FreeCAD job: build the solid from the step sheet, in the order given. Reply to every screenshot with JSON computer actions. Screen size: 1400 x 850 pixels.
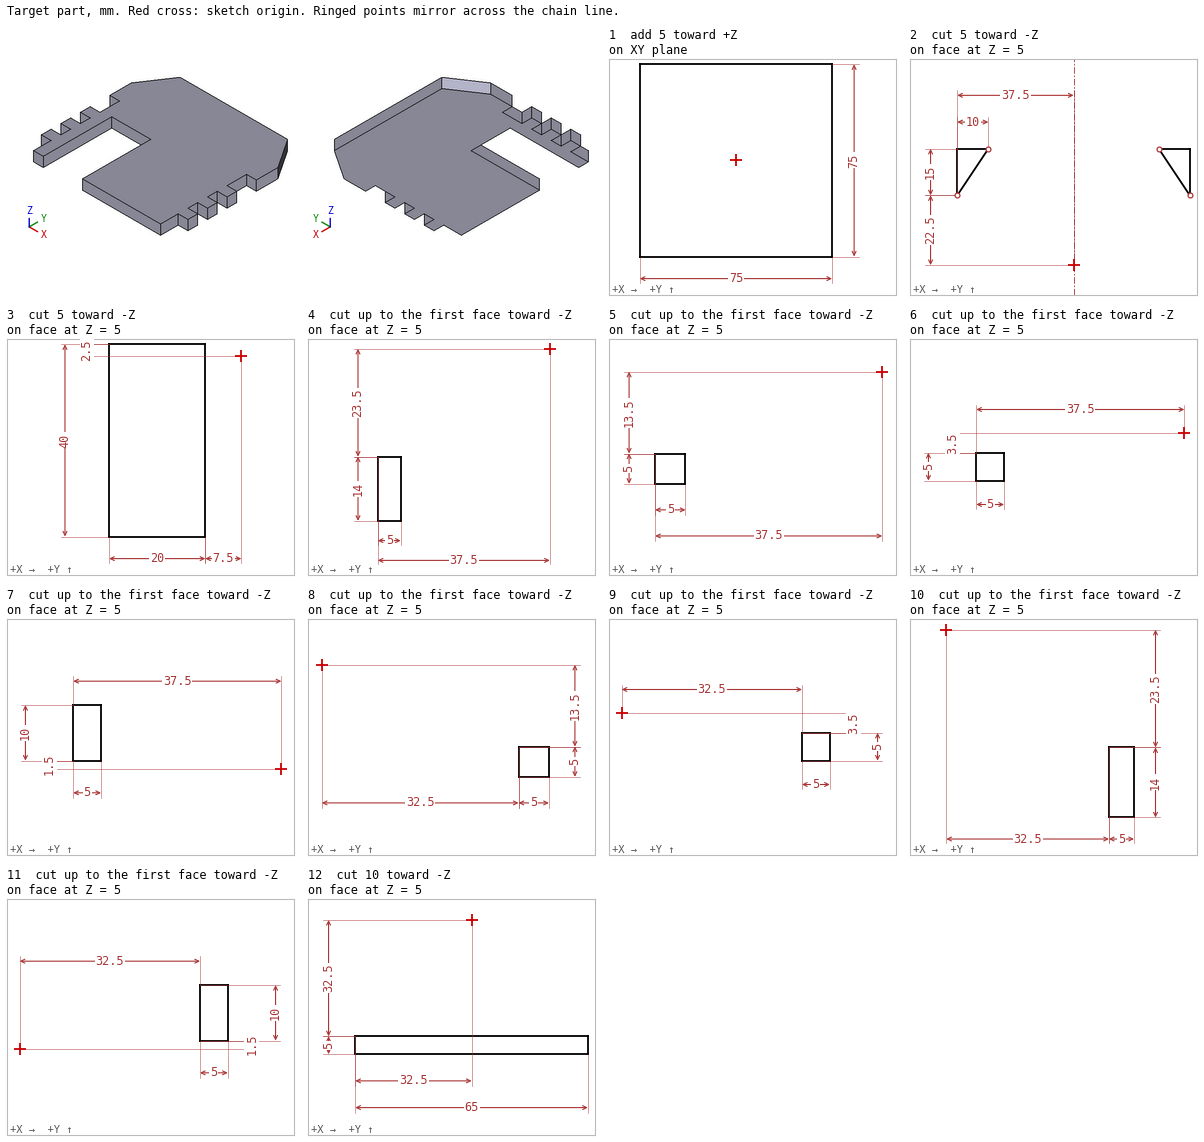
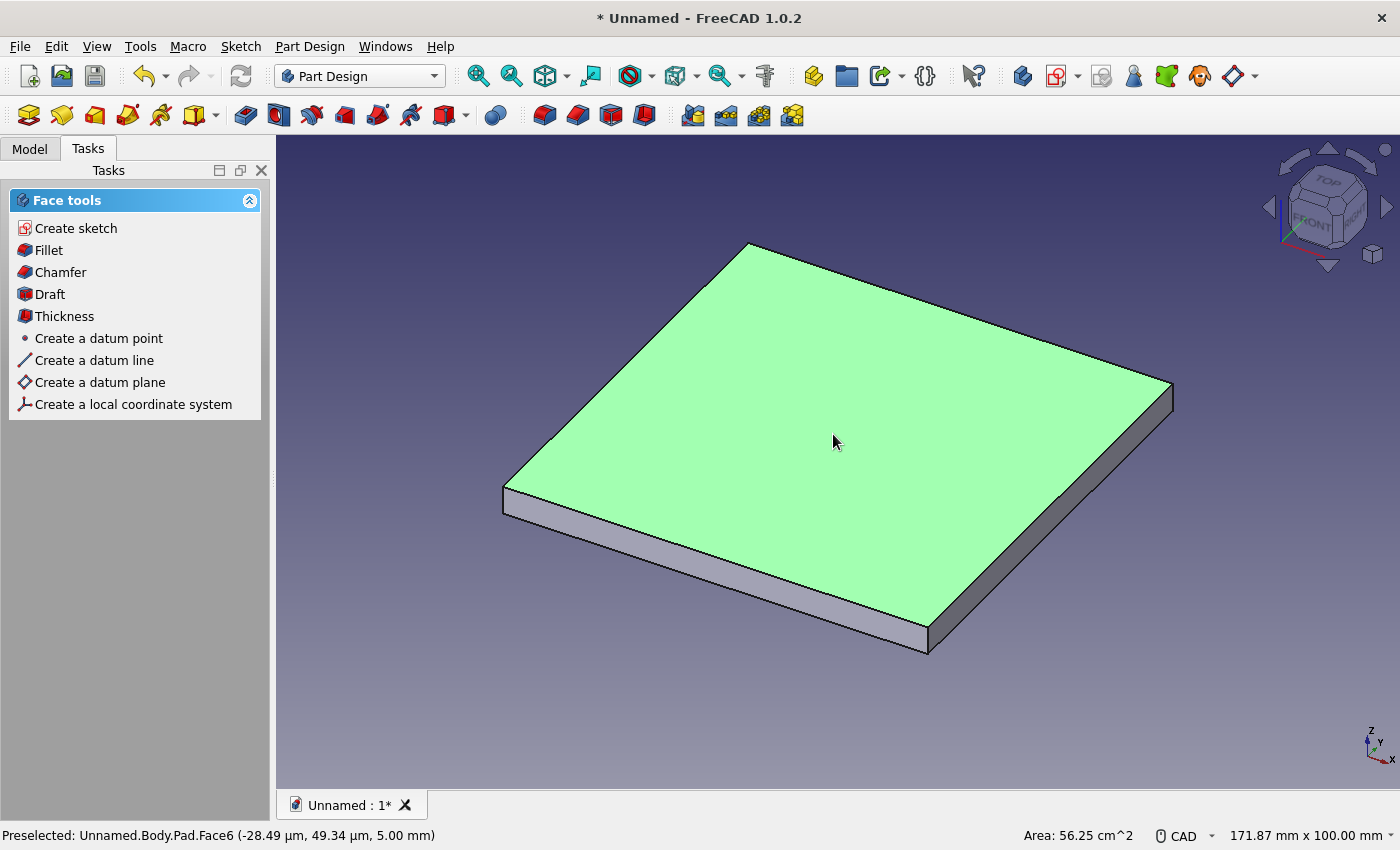
{"action": "left_click", "coordinate": [1056, 76]}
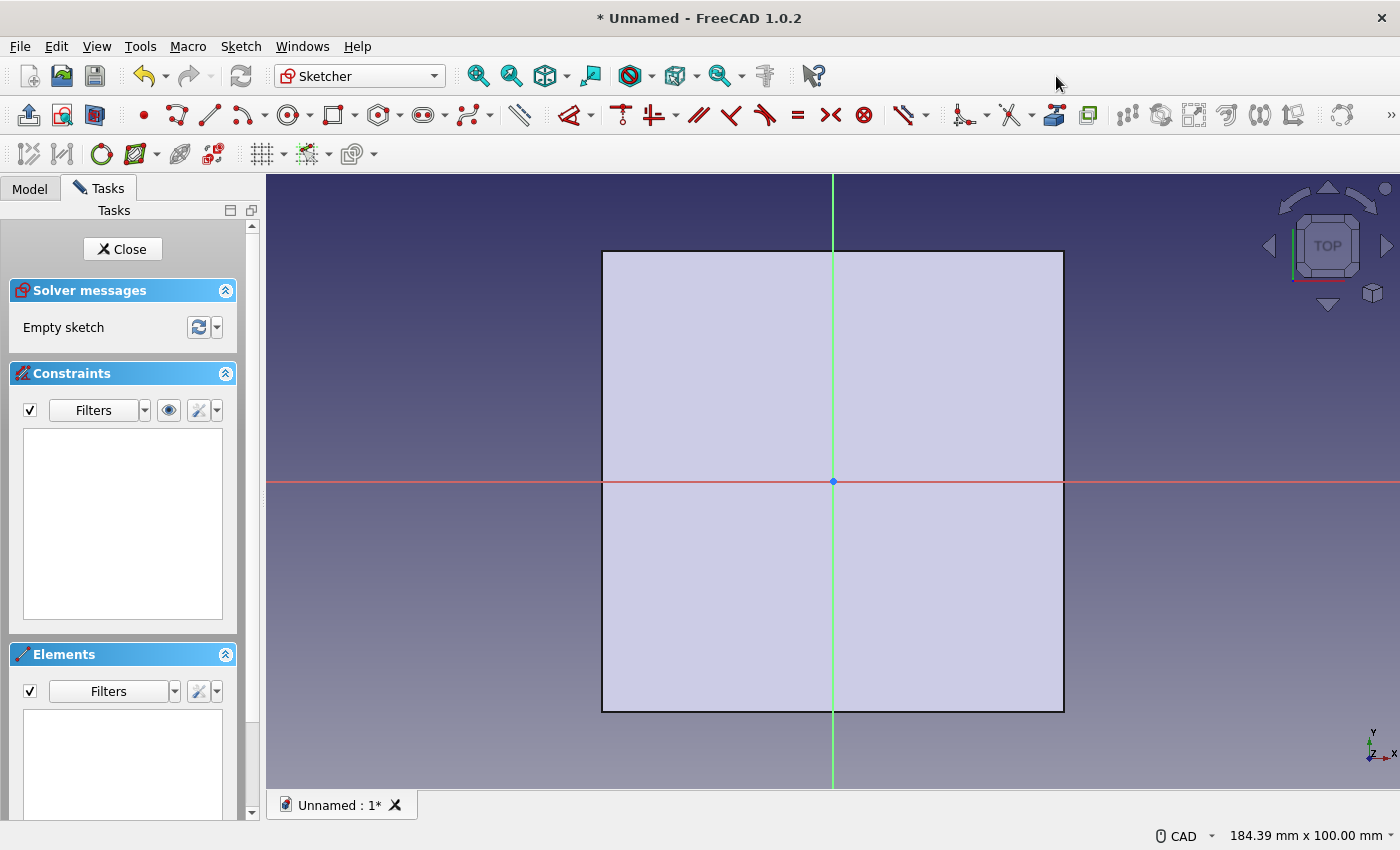
{"action": "scroll", "coordinate": [972, 202], "scroll_direction": "up", "scroll_amount": 2}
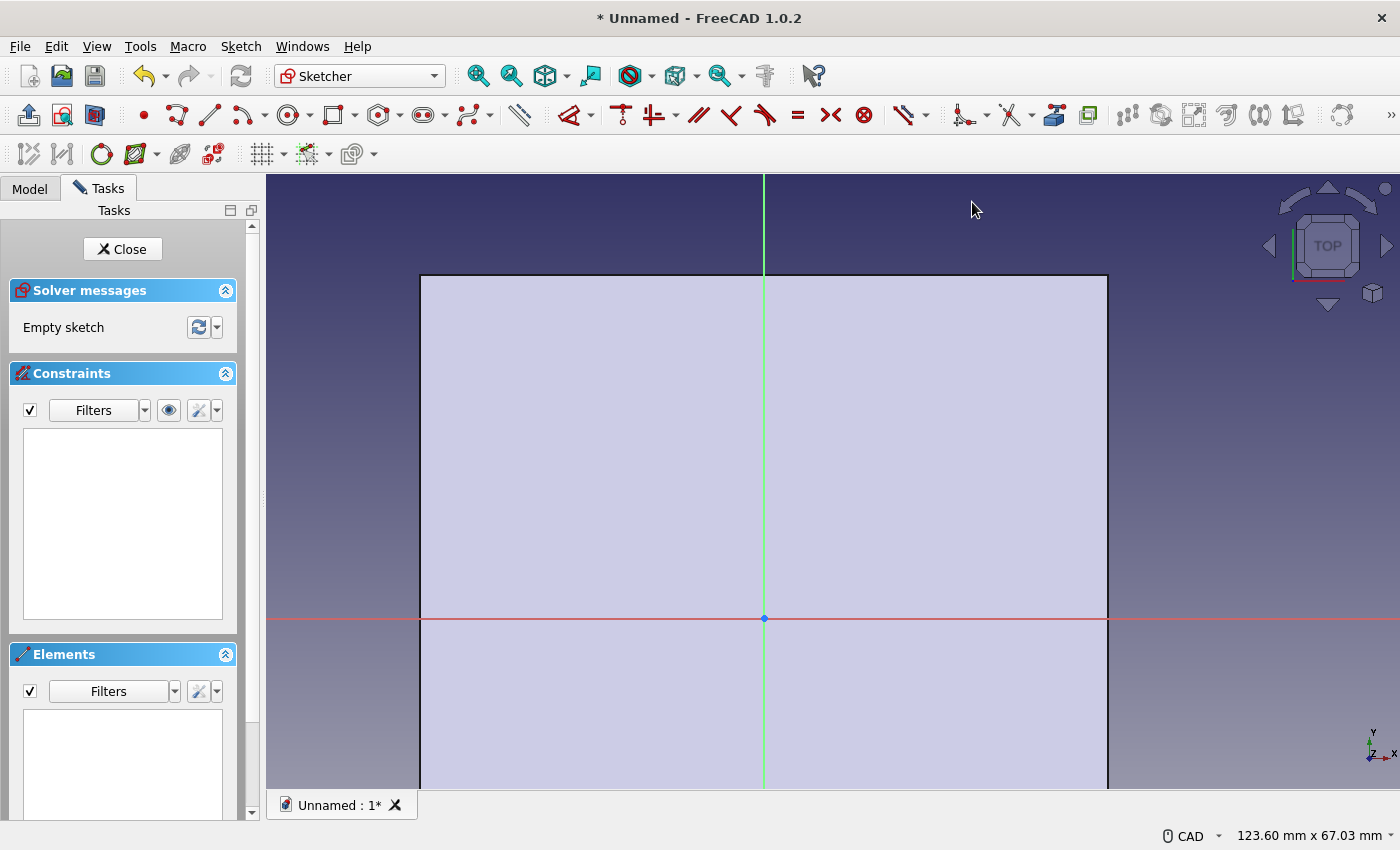
{"action": "left_click", "coordinate": [177, 116]}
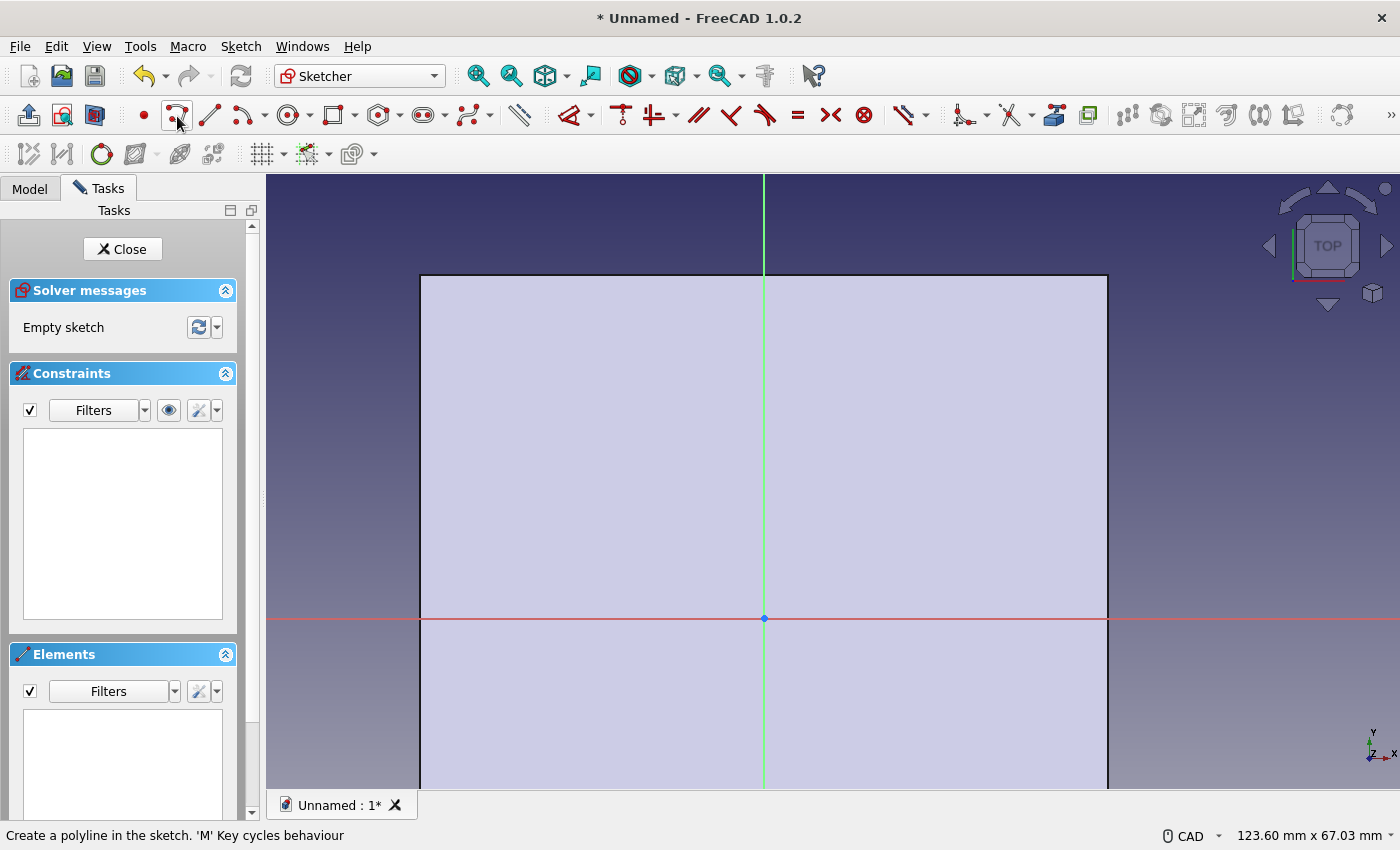
{"action": "left_click", "coordinate": [420, 413]}
{"action": "left_click", "coordinate": [512, 275]}
{"action": "left_click", "coordinate": [420, 275]}
{"action": "left_click", "coordinate": [420, 414]}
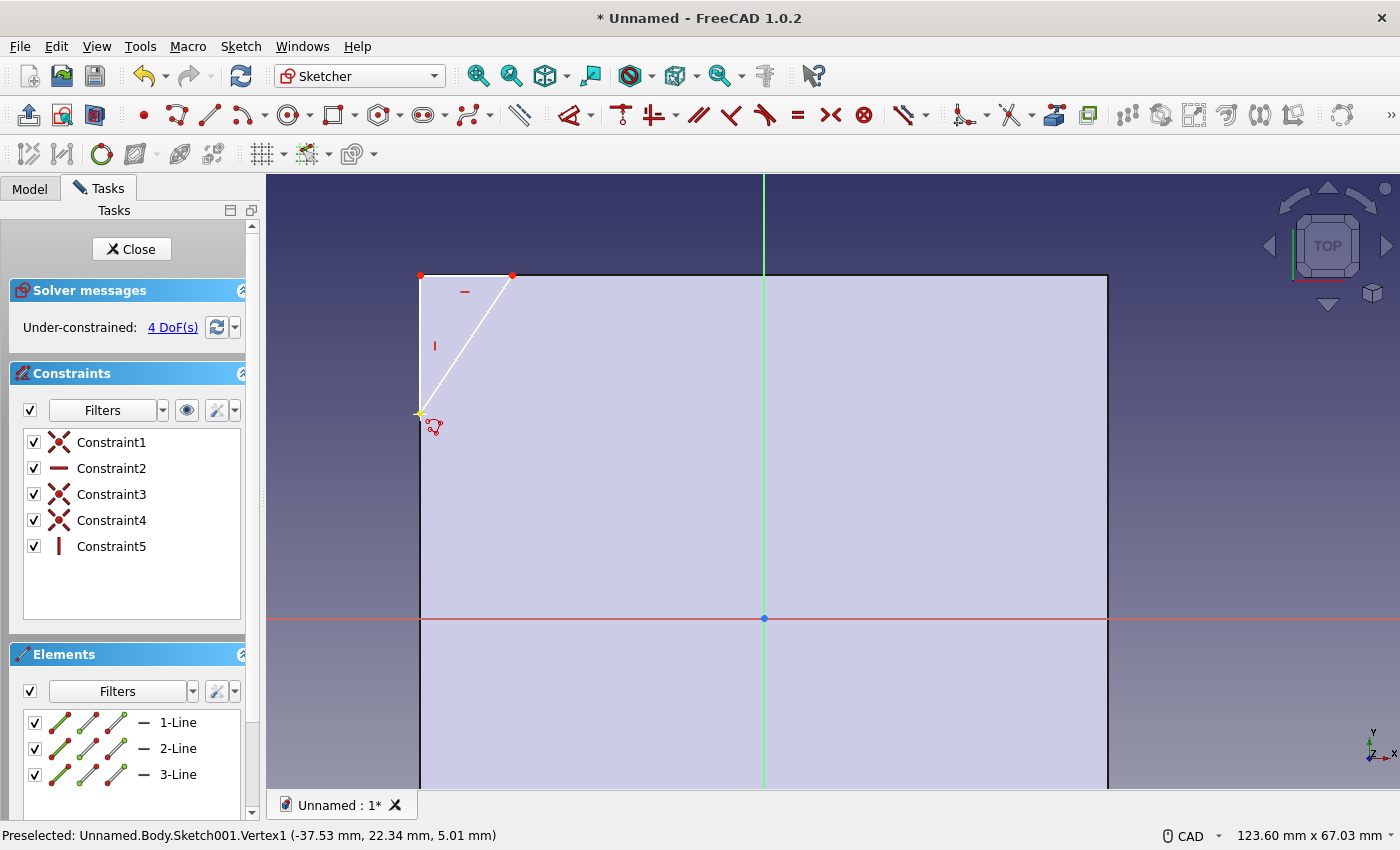
{"action": "left_click", "coordinate": [1108, 413]}
{"action": "left_click", "coordinate": [1108, 275]}
{"action": "left_click", "coordinate": [1017, 275]}
{"action": "left_click", "coordinate": [1108, 414]}
{"action": "key", "text": "Escape"}
{"action": "key", "text": "Escape"}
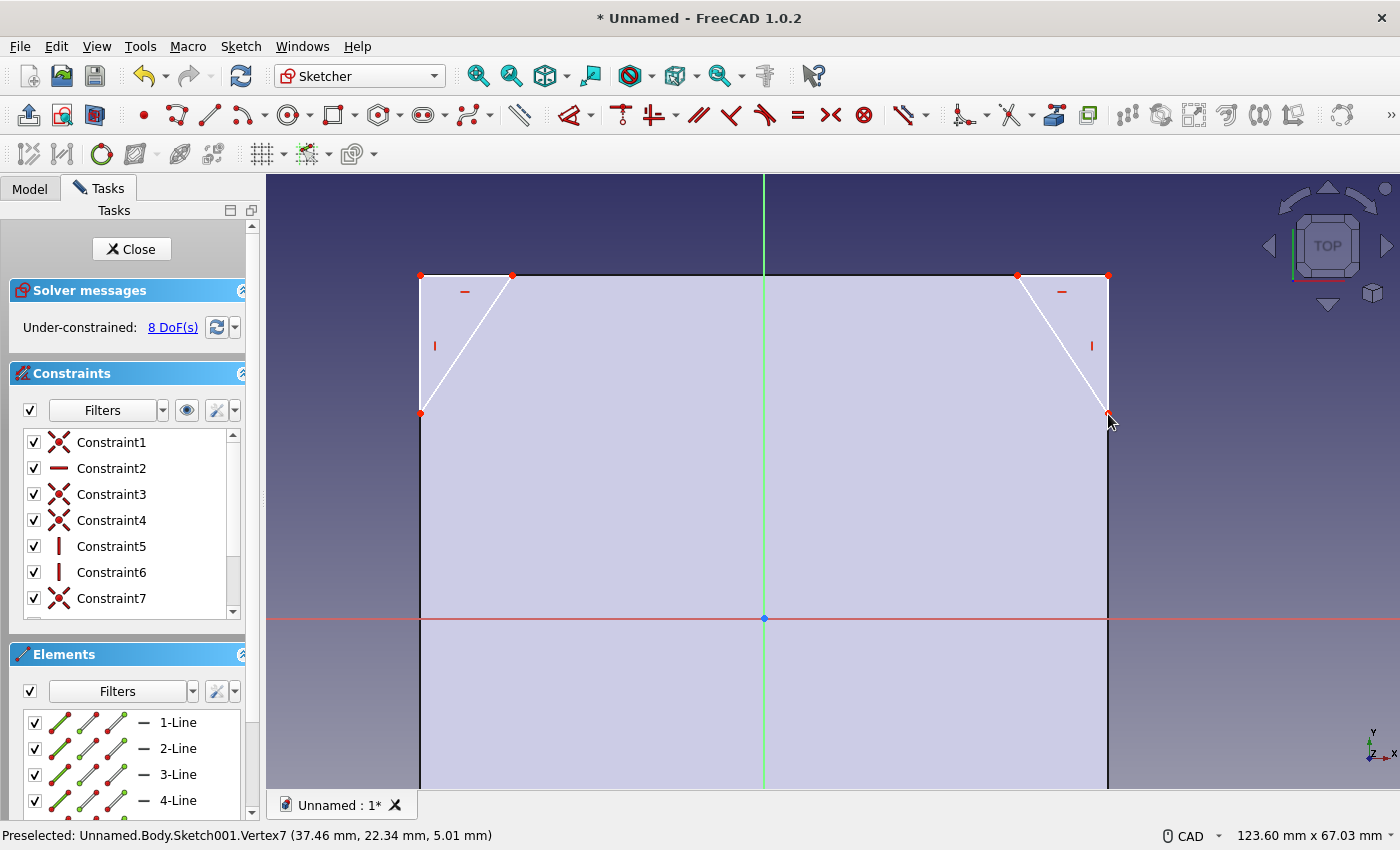
{"action": "left_click", "coordinate": [420, 414]}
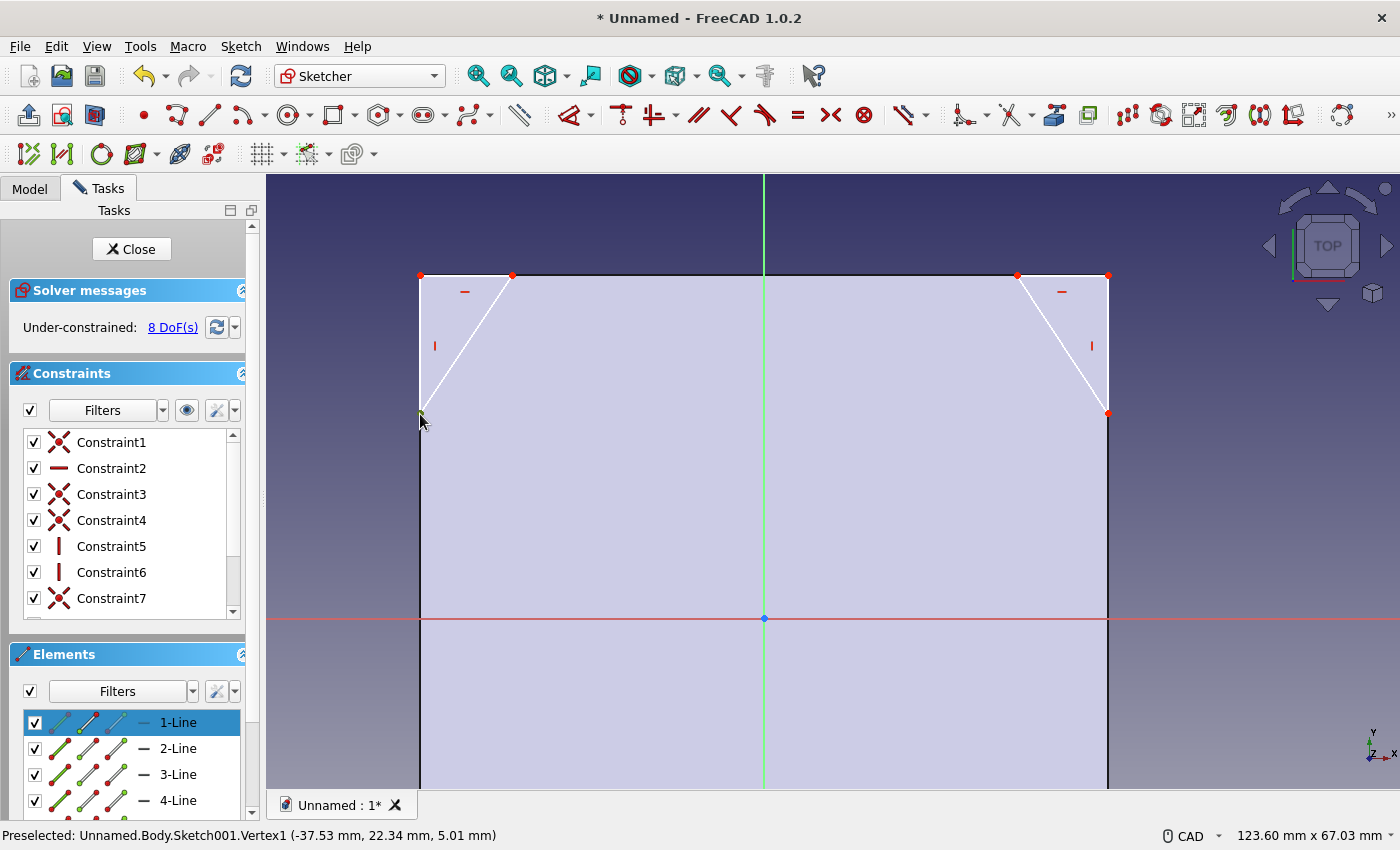
{"action": "left_click", "coordinate": [1108, 414]}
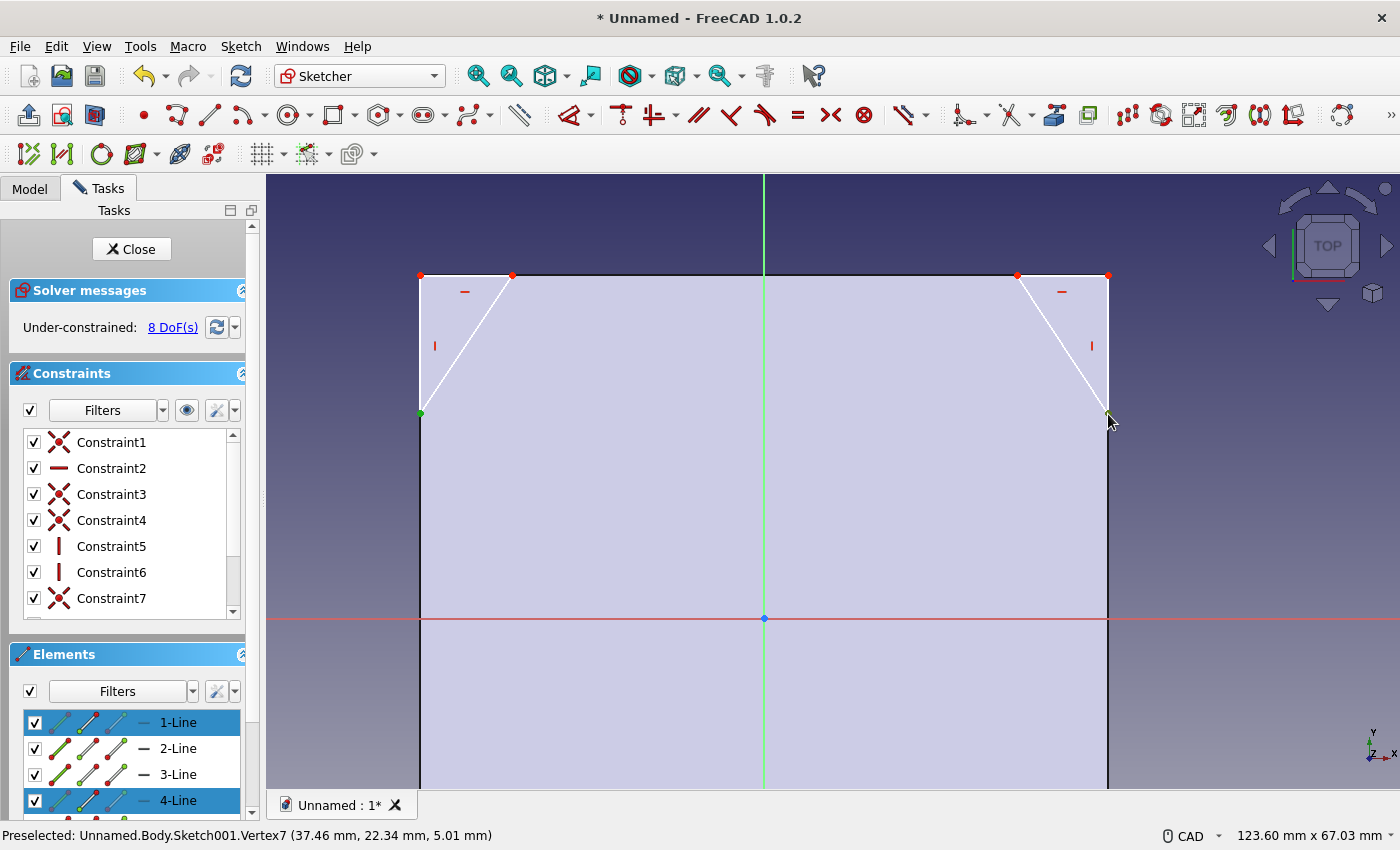
{"action": "left_click", "coordinate": [764, 721]}